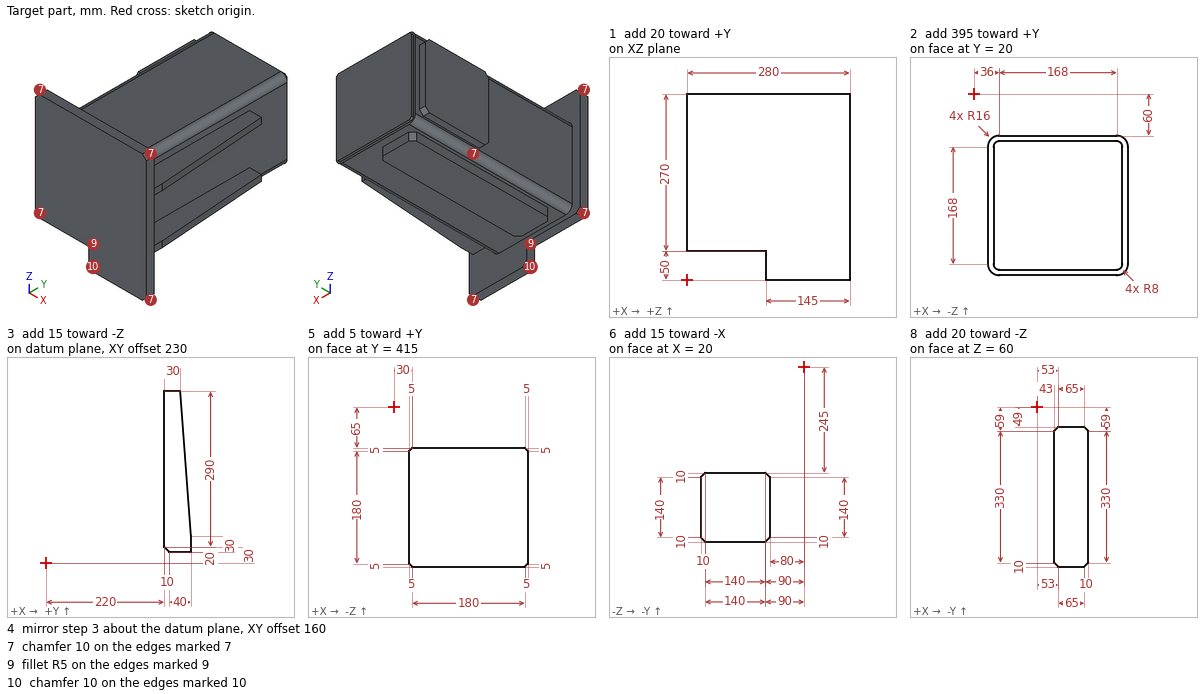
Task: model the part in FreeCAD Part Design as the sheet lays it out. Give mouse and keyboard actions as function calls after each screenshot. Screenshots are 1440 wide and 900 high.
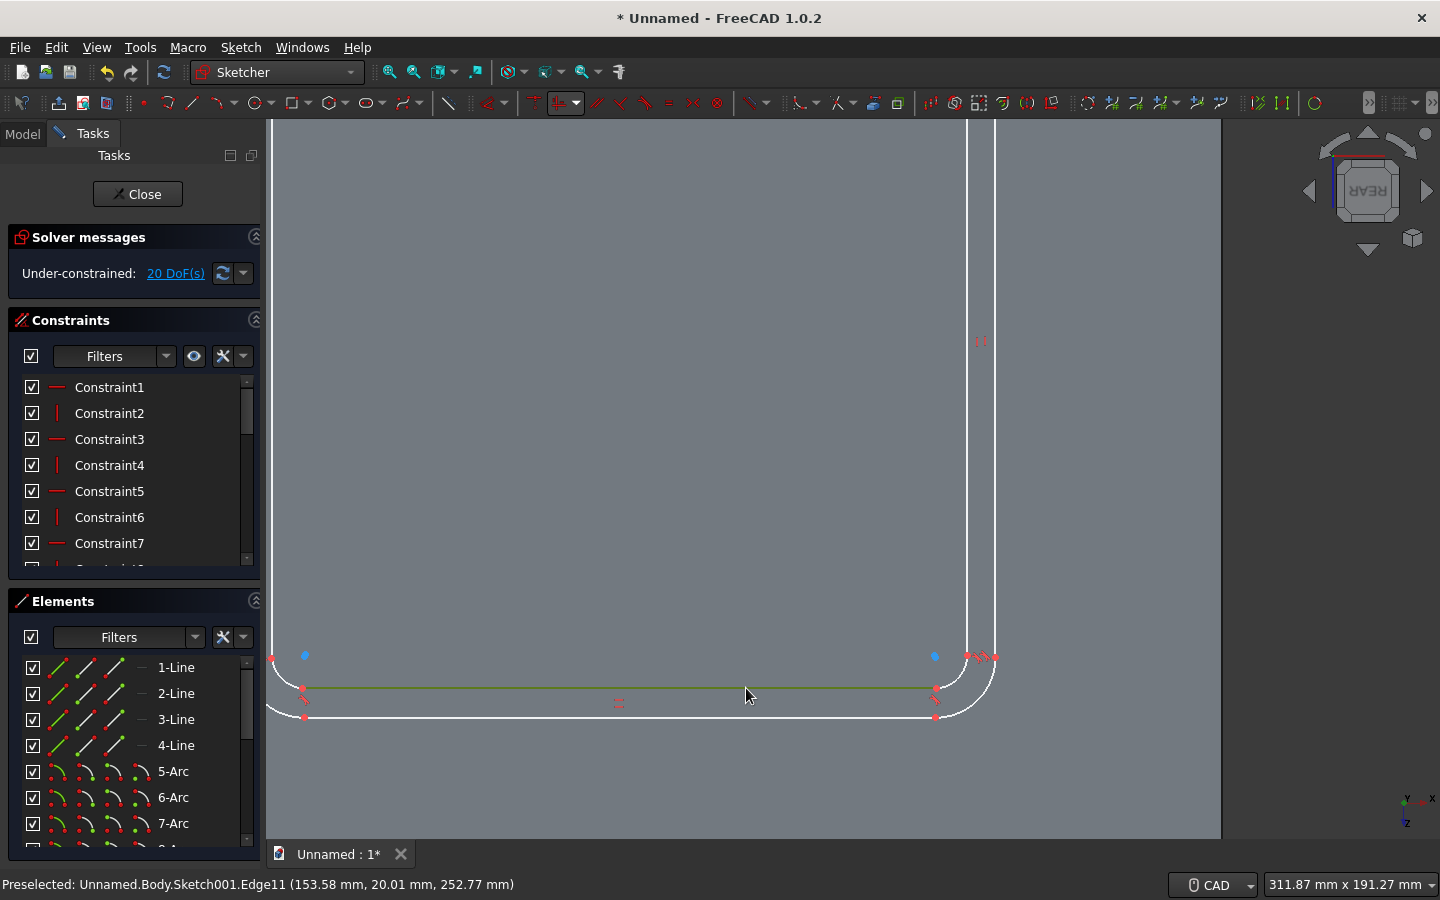
click(951, 684)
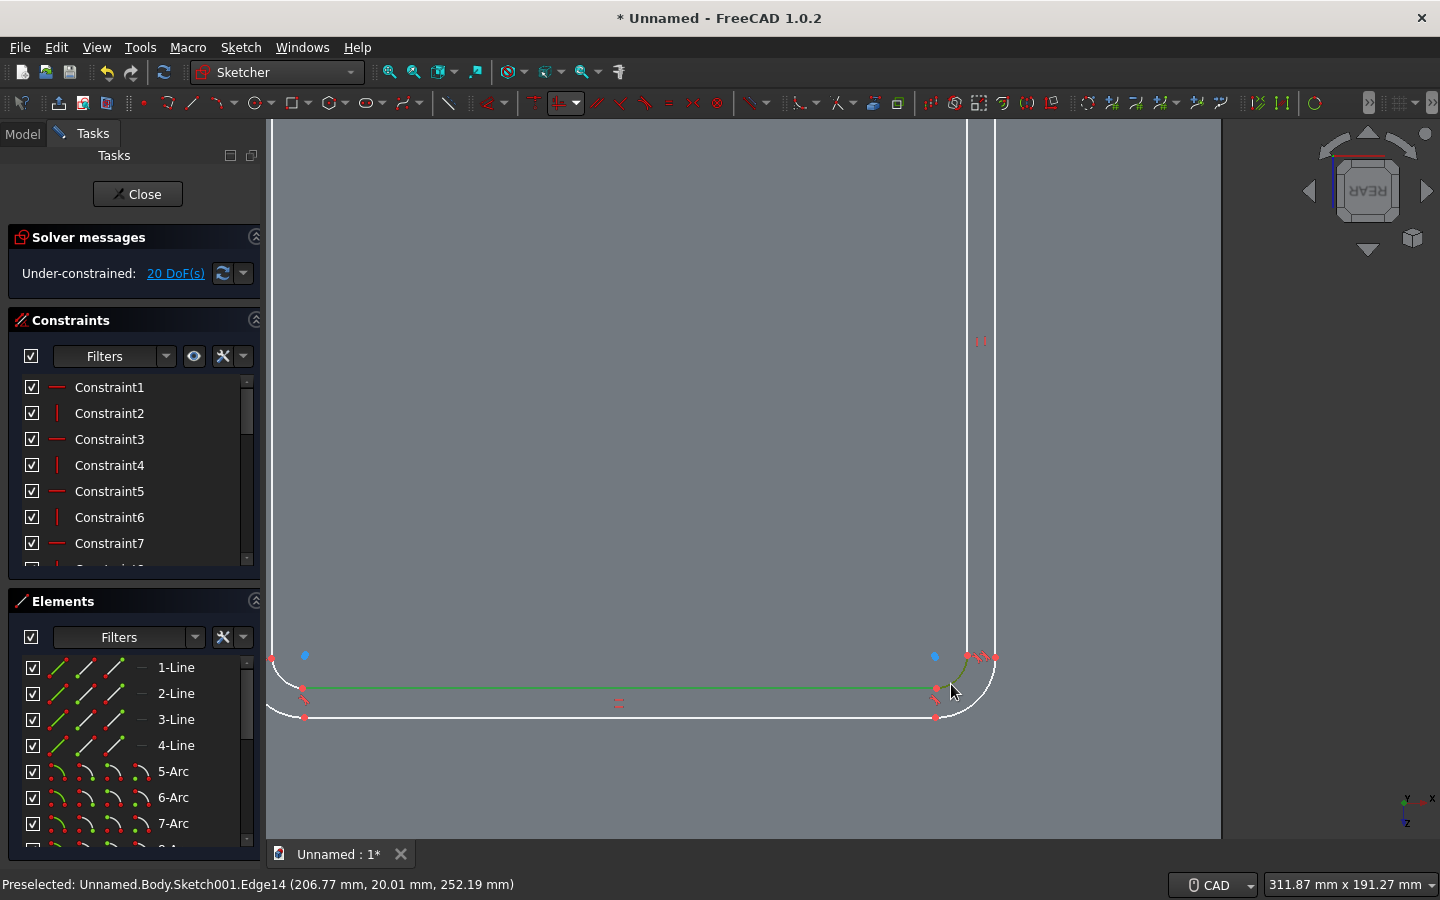
key(t)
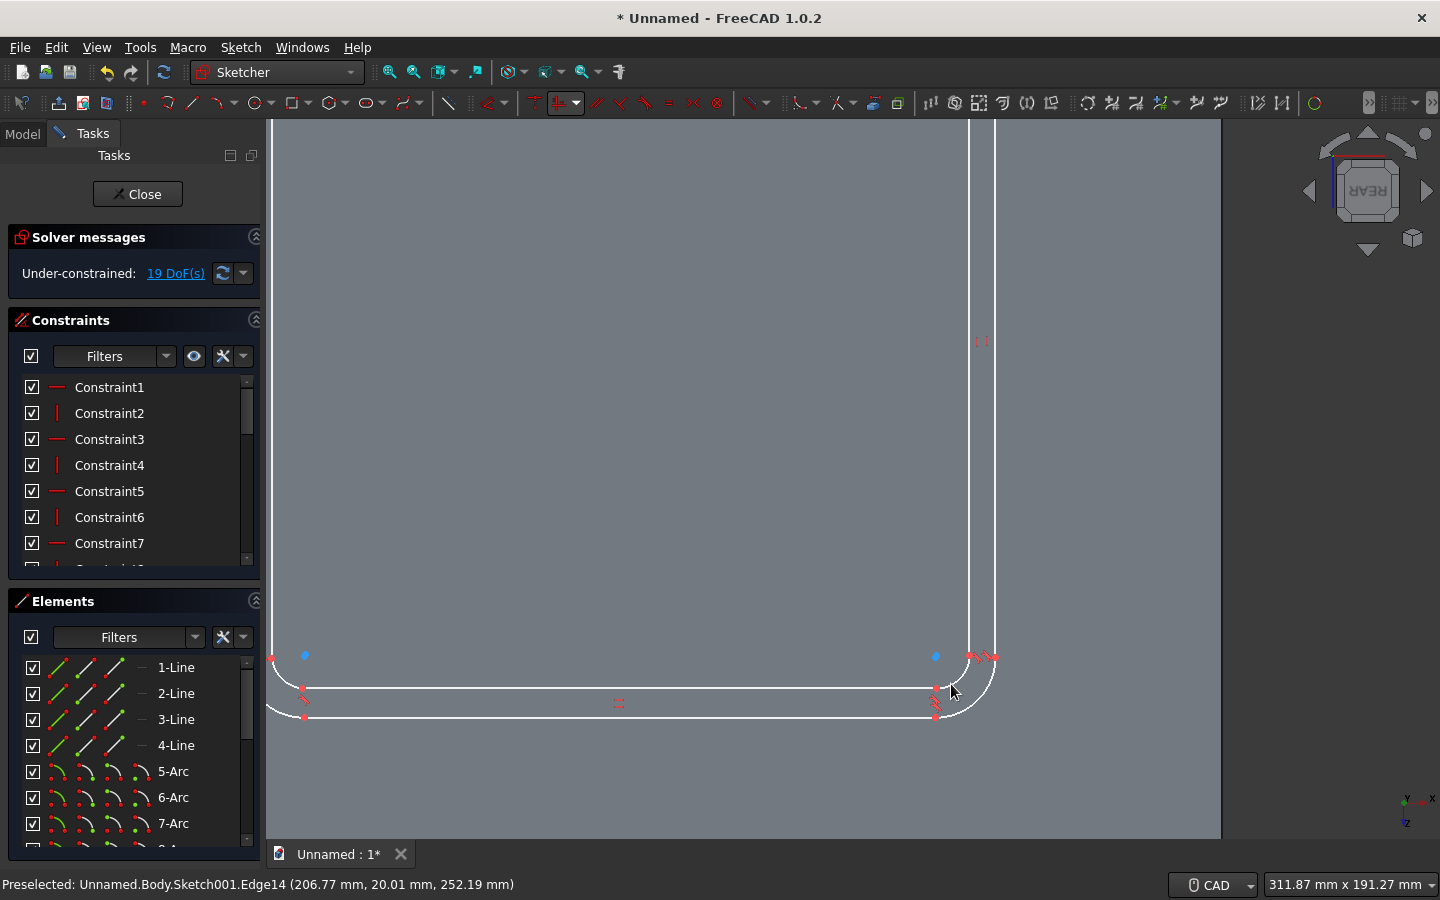
click(746, 688)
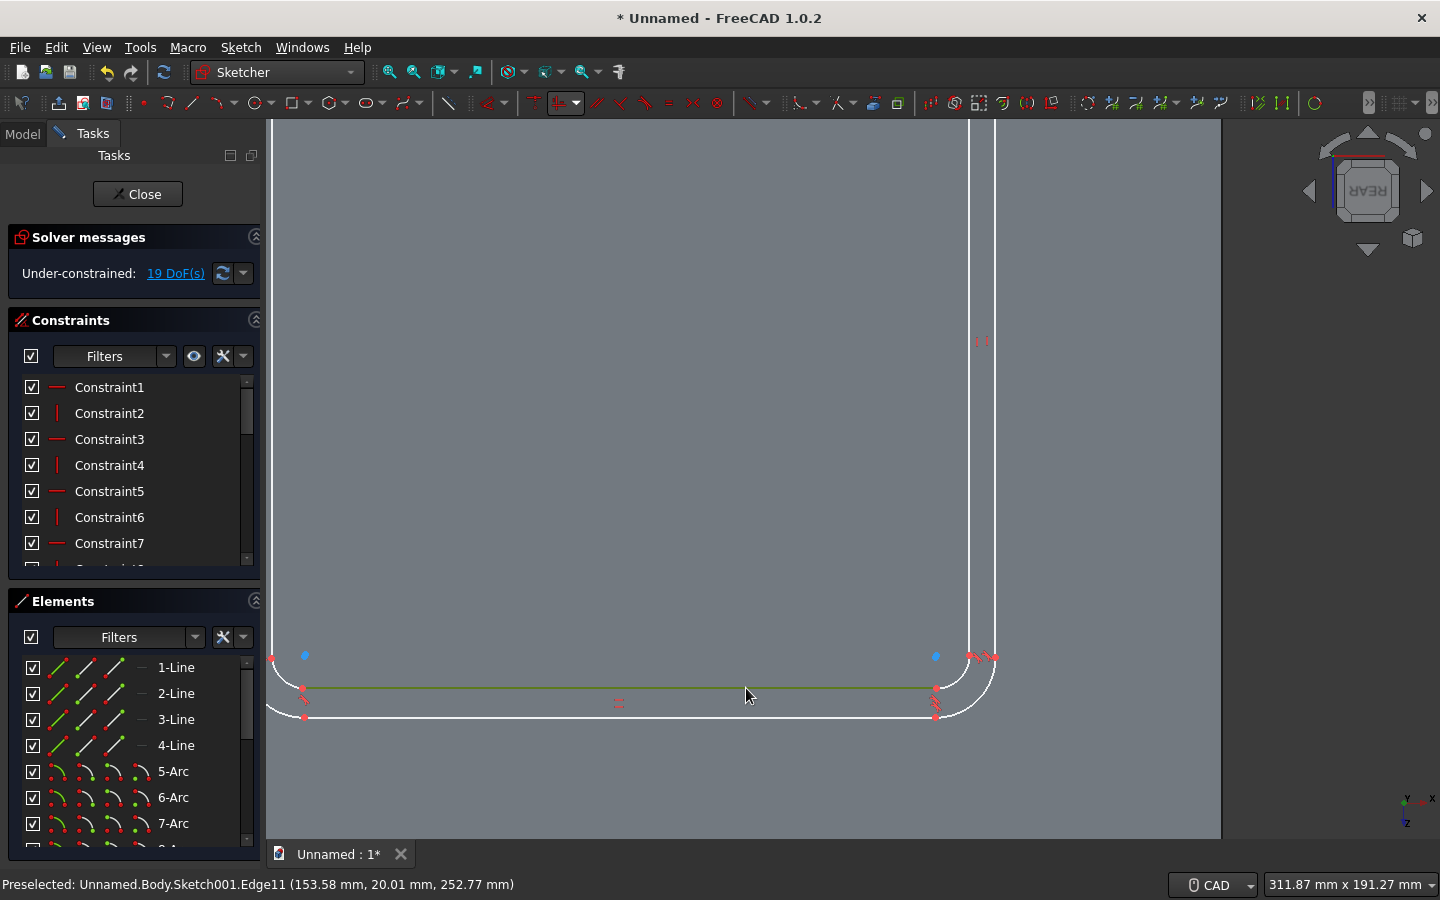
scroll(950, 685, down, 4)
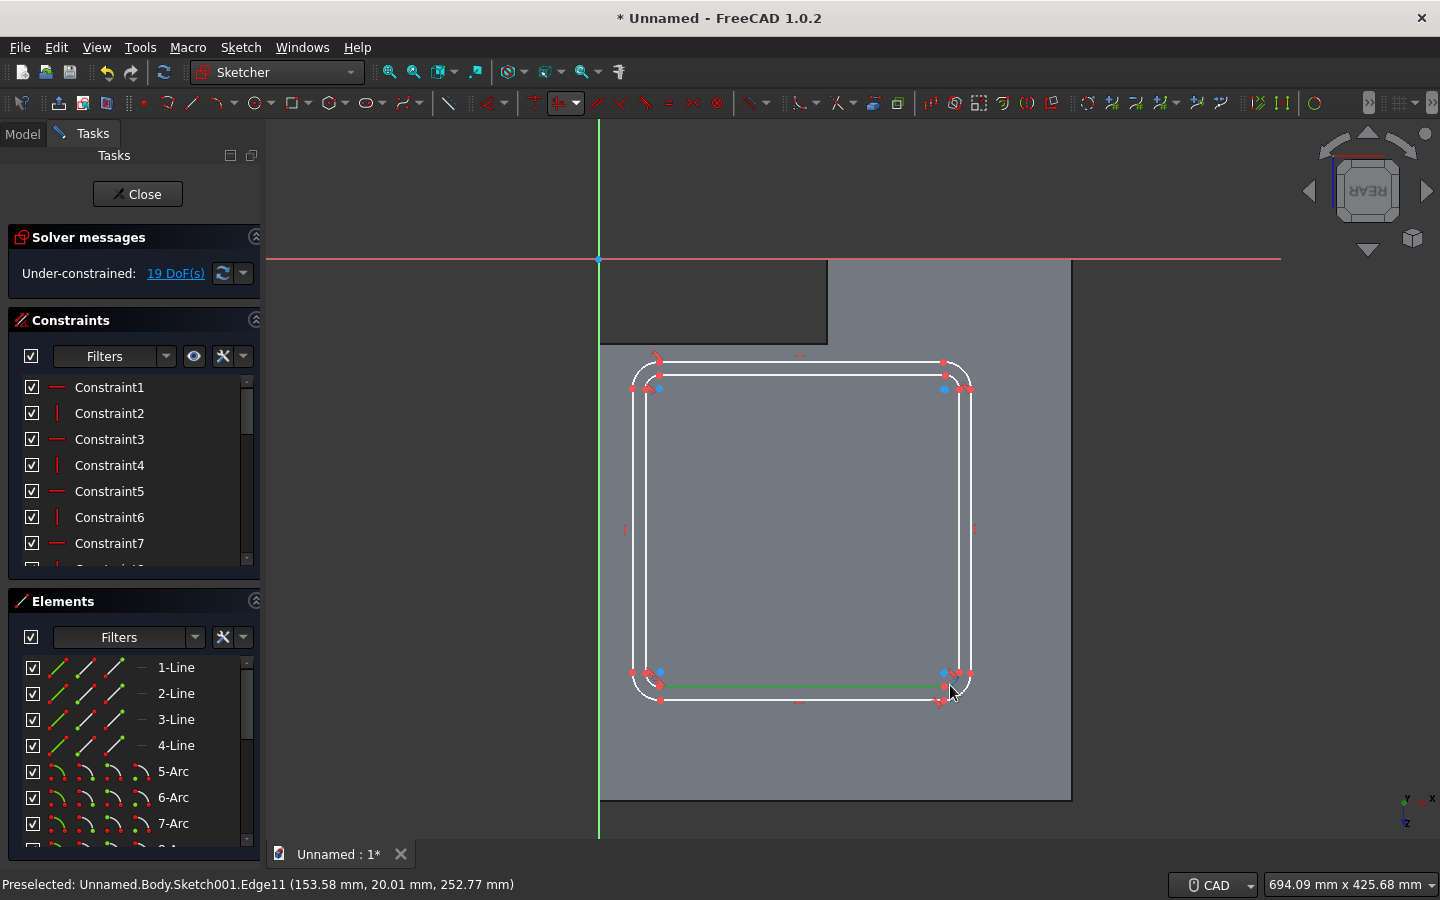
scroll(648, 679, up, 4)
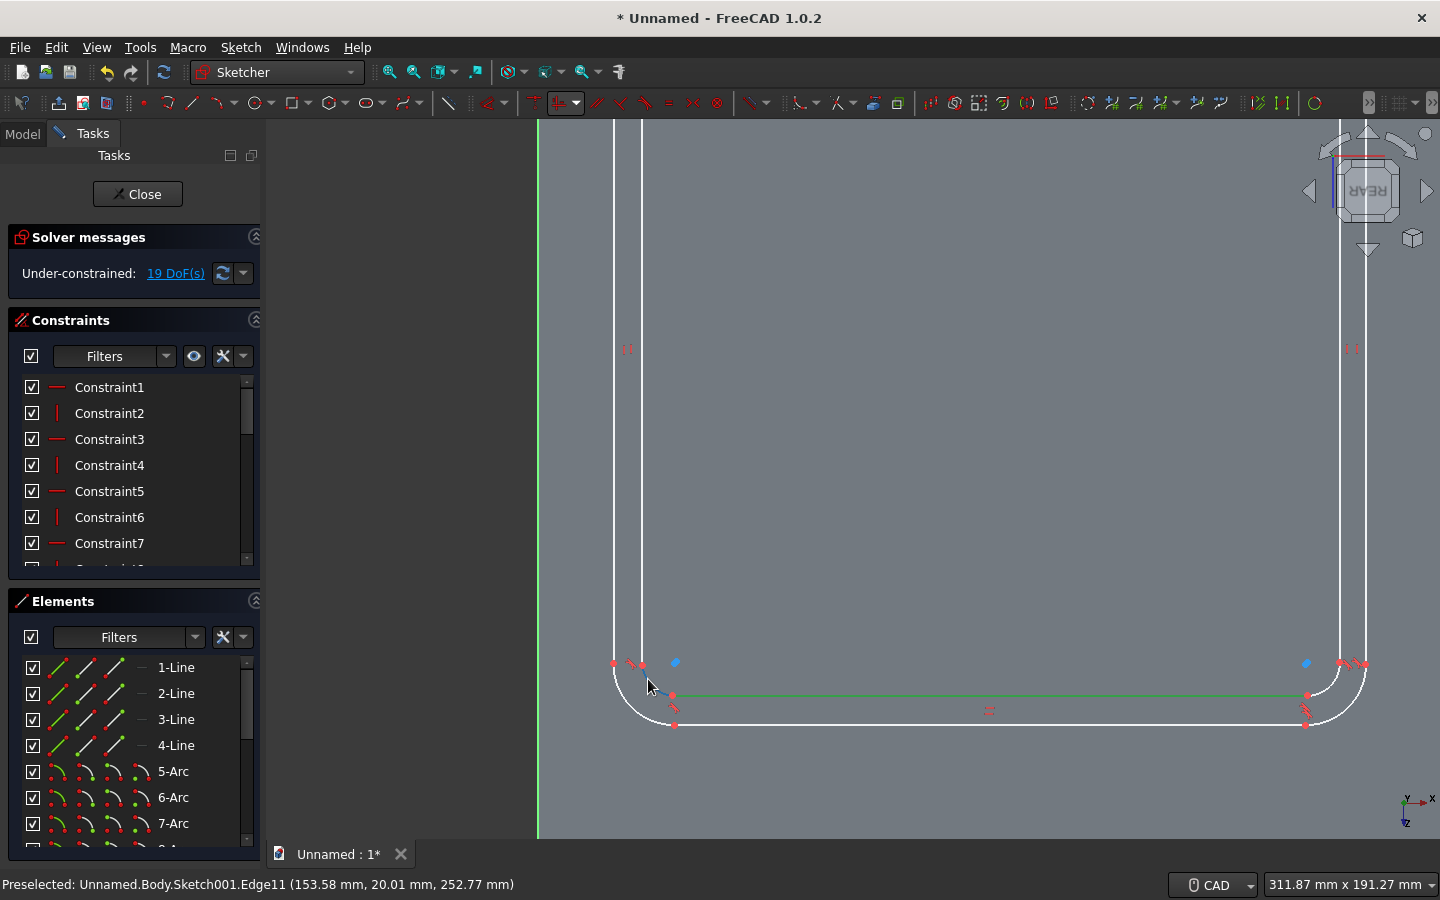
click(647, 679)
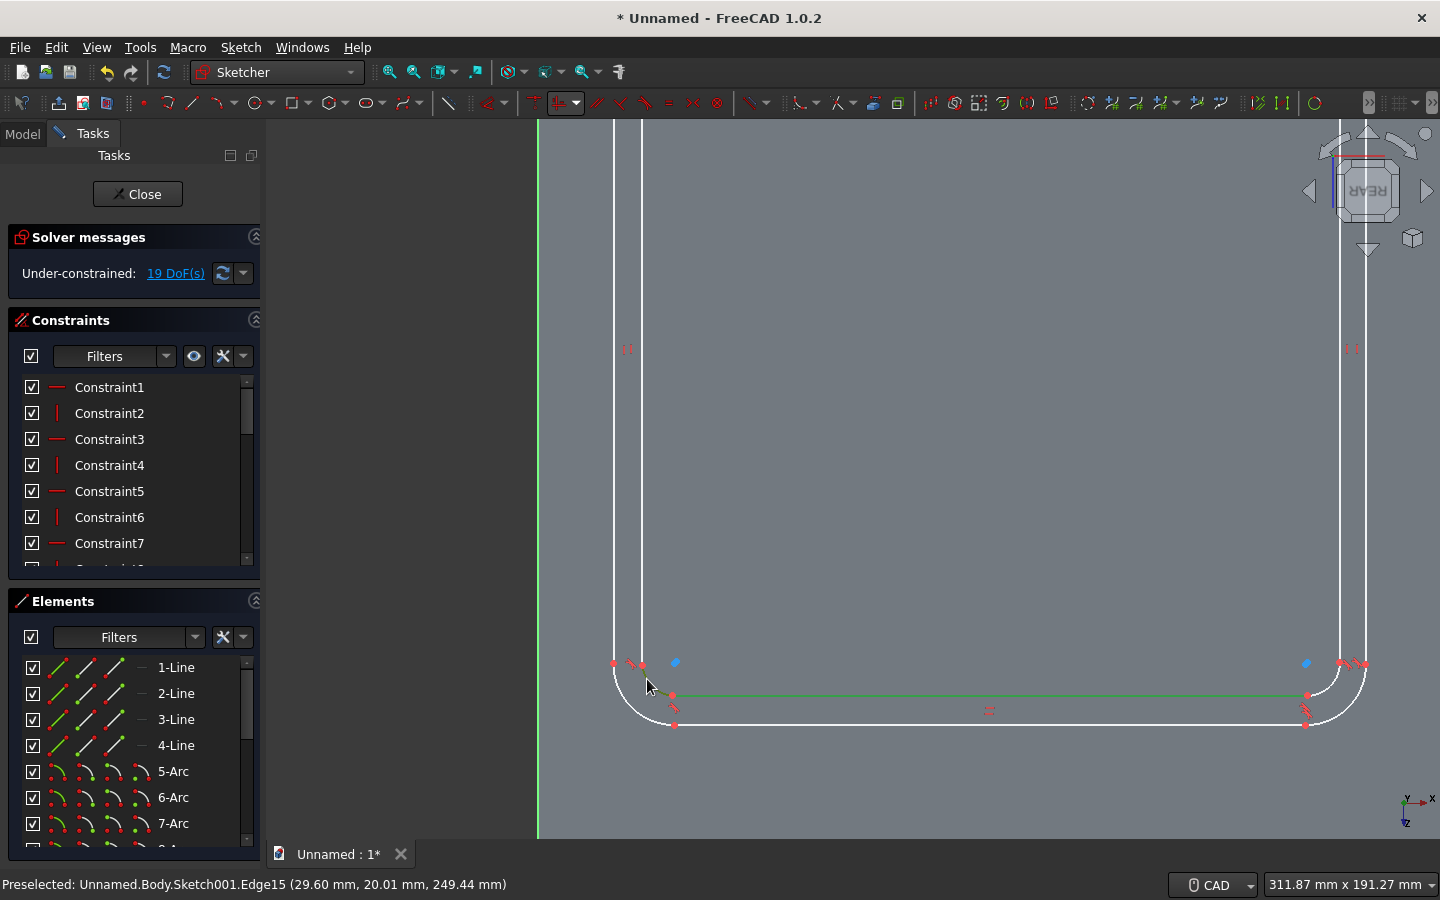
click(646, 104)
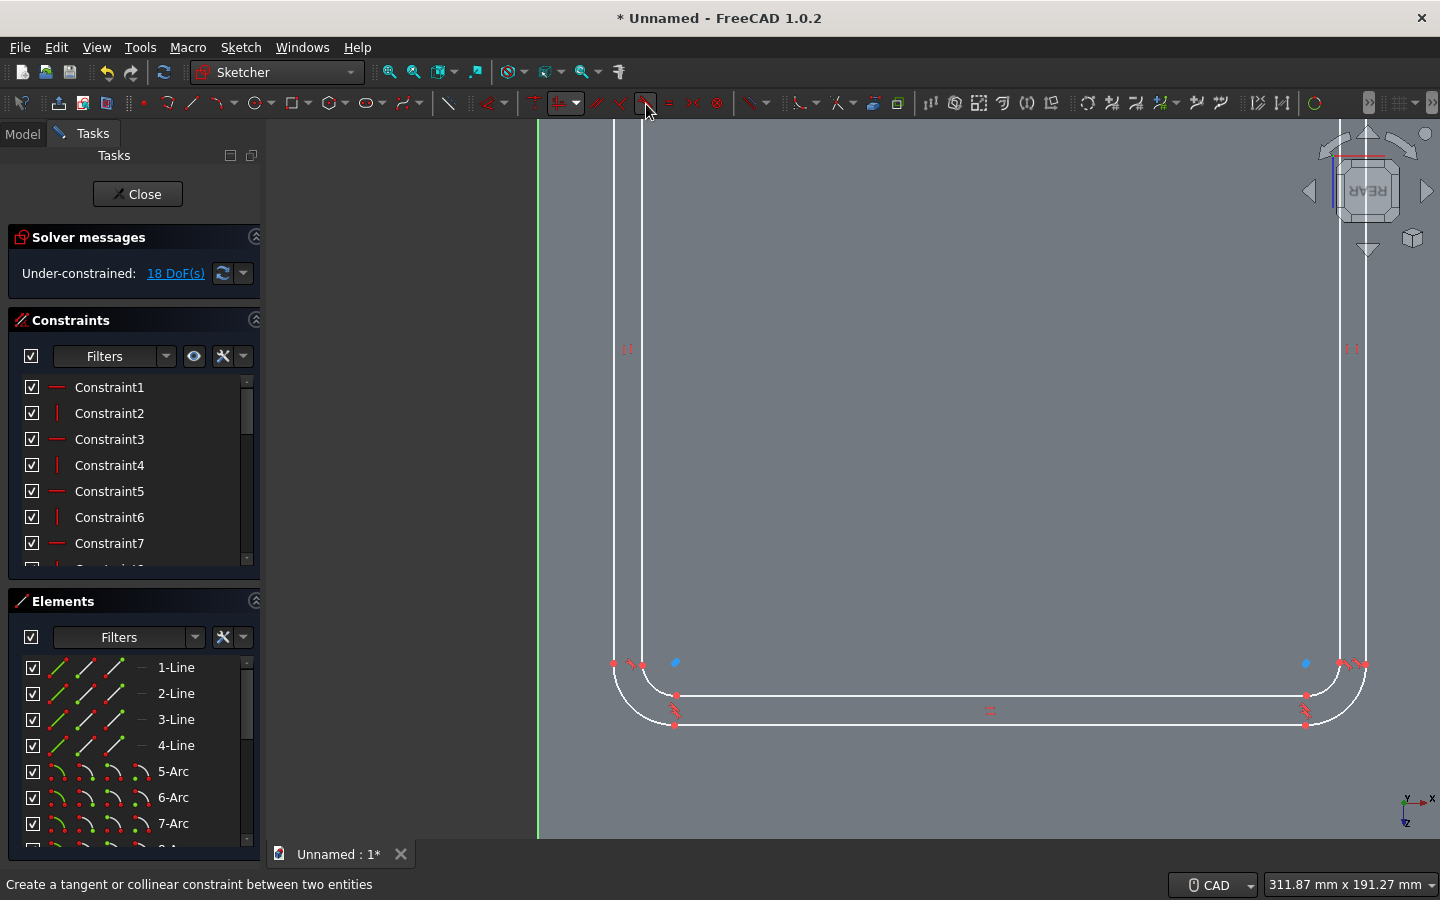
click(642, 476)